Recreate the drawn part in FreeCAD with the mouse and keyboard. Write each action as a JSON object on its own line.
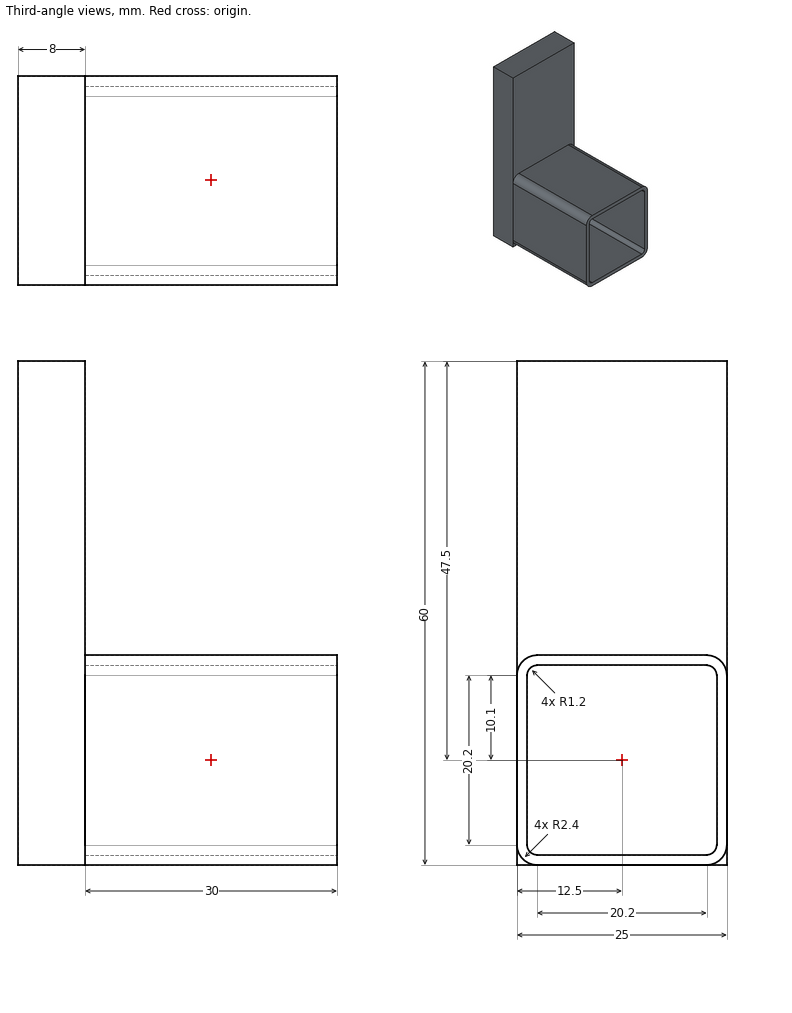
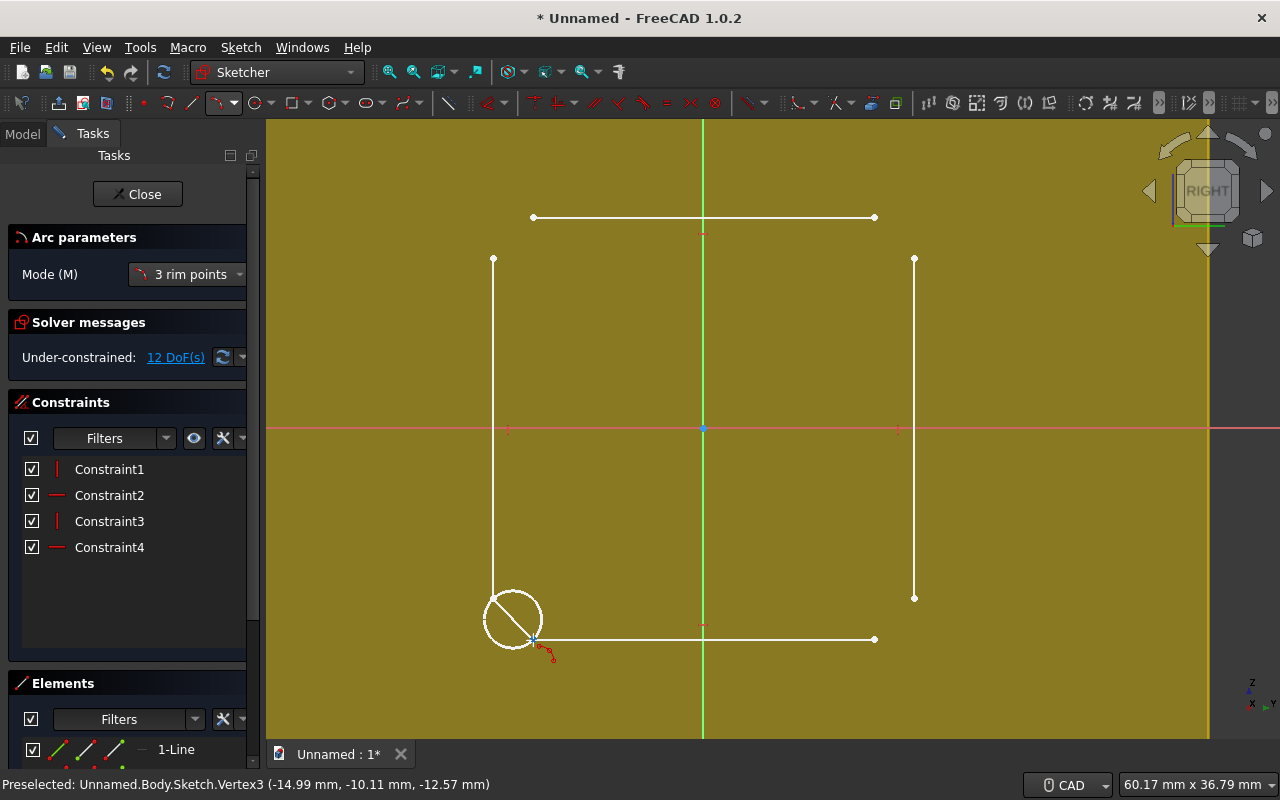
{"action": "scroll", "coordinate": [505, 627], "scroll_direction": "up", "scroll_amount": 2}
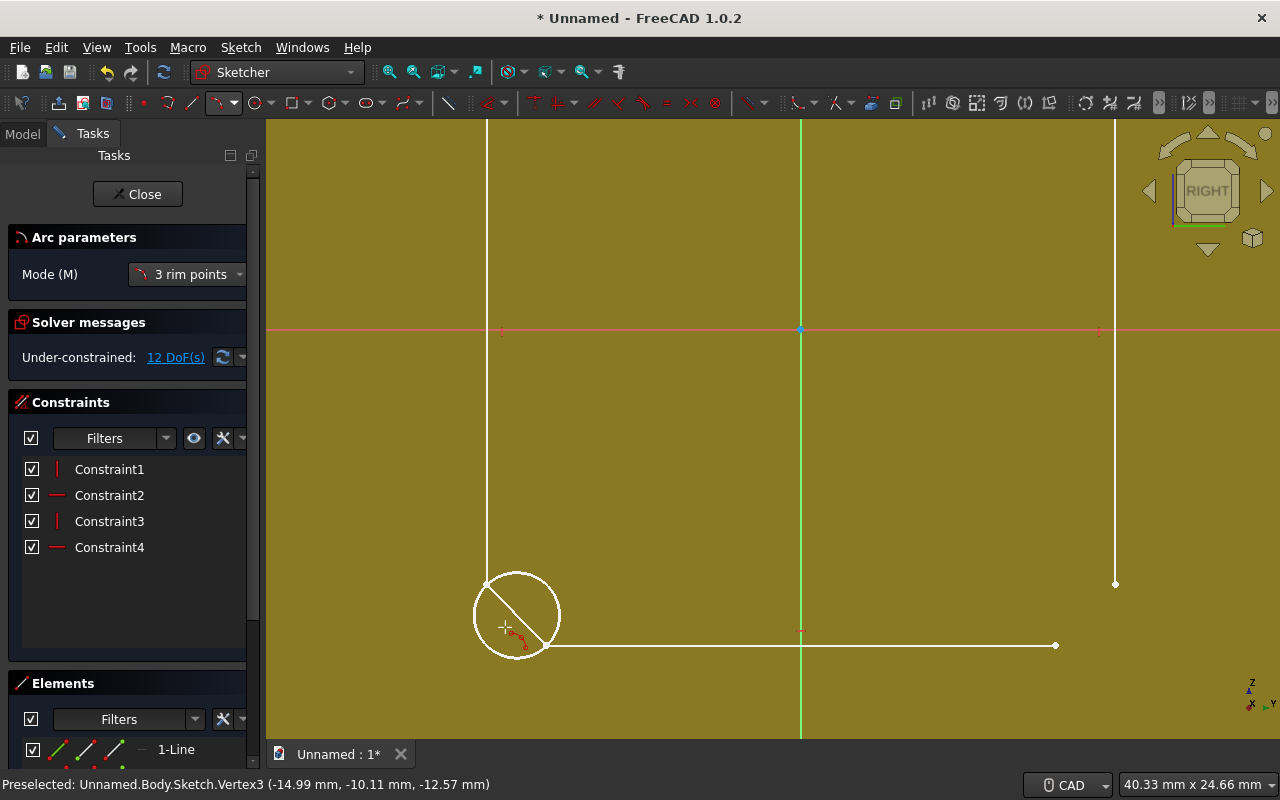
{"action": "left_click", "coordinate": [504, 627]}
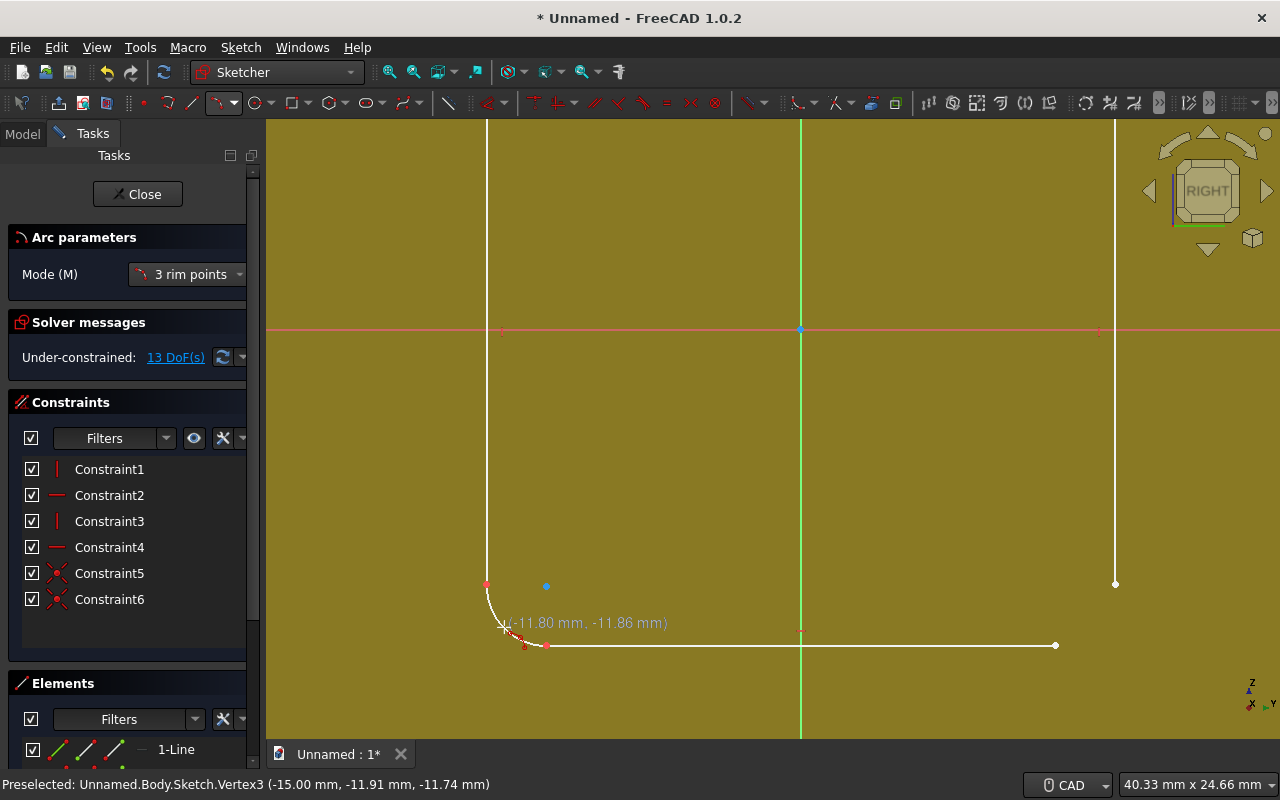
{"action": "left_click", "coordinate": [1055, 646]}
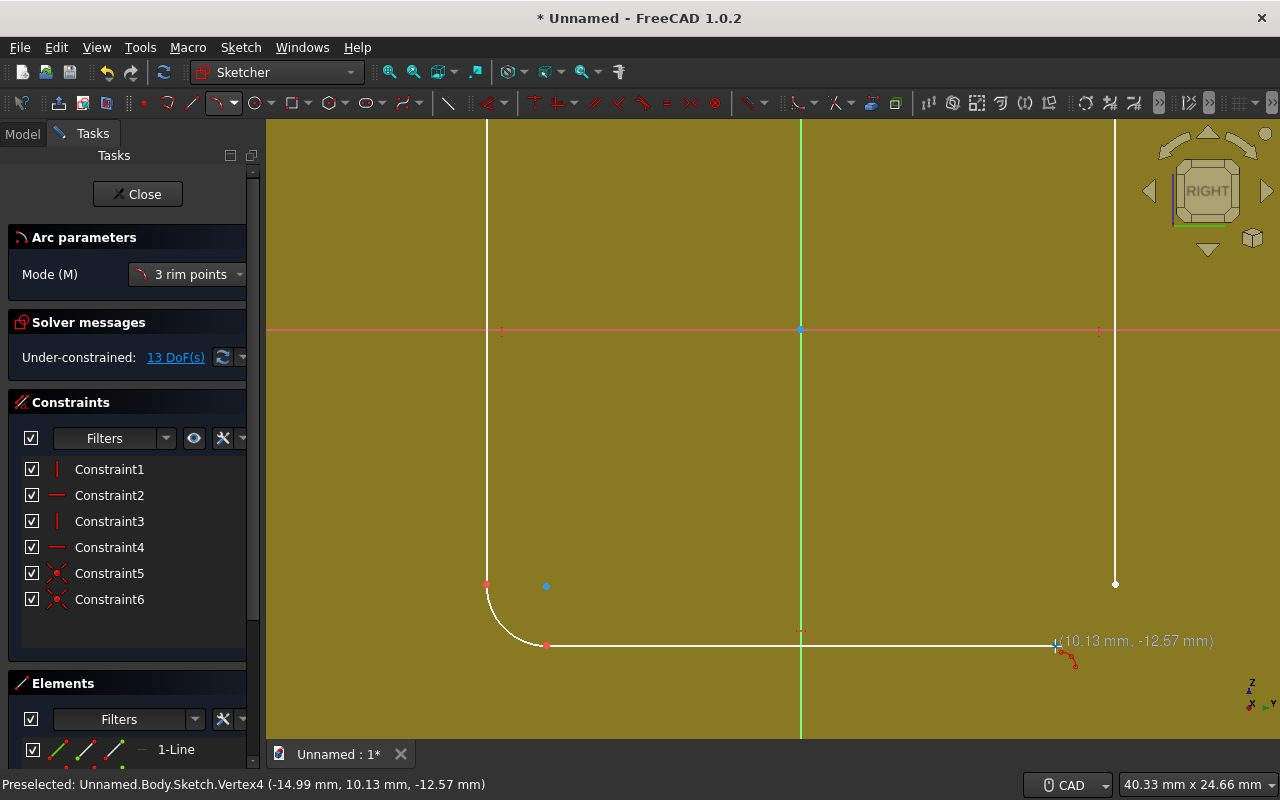
{"action": "scroll", "coordinate": [509, 630], "scroll_direction": "down", "scroll_amount": 2}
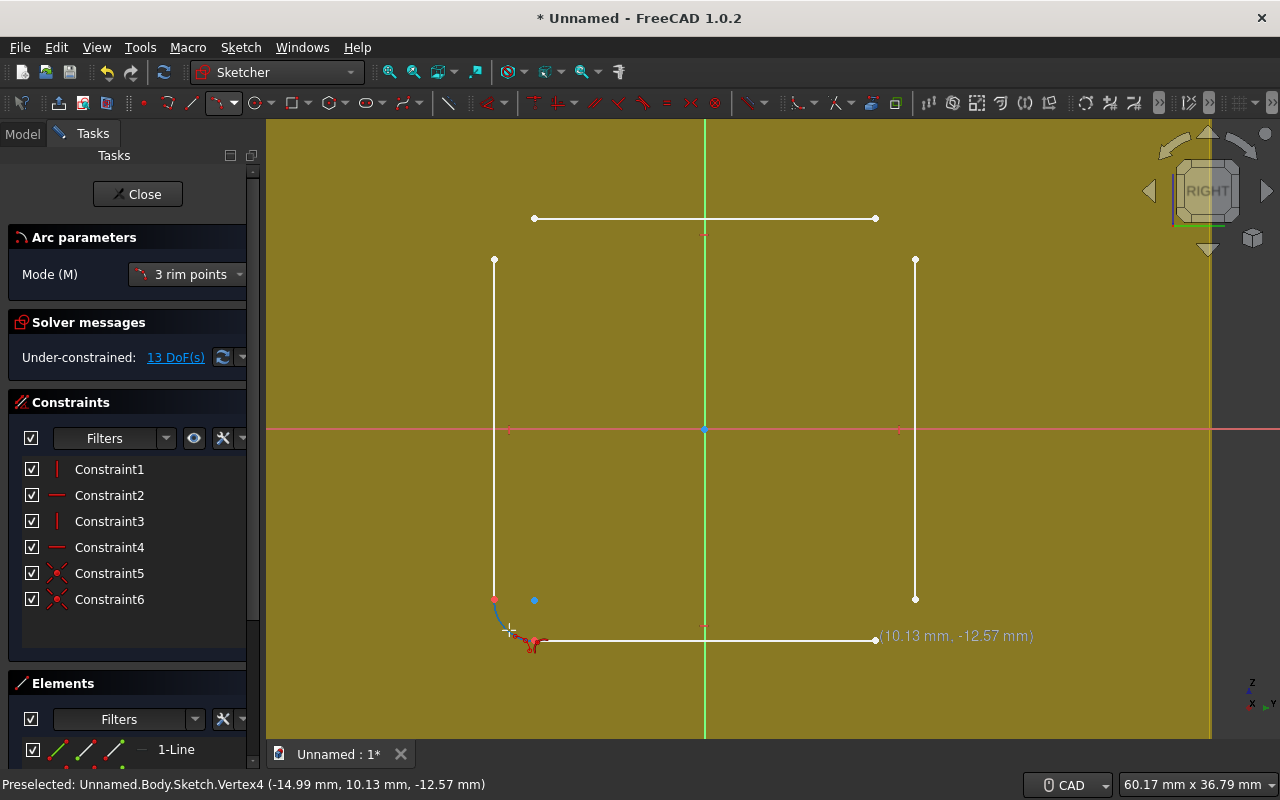
{"action": "left_click", "coordinate": [915, 600]}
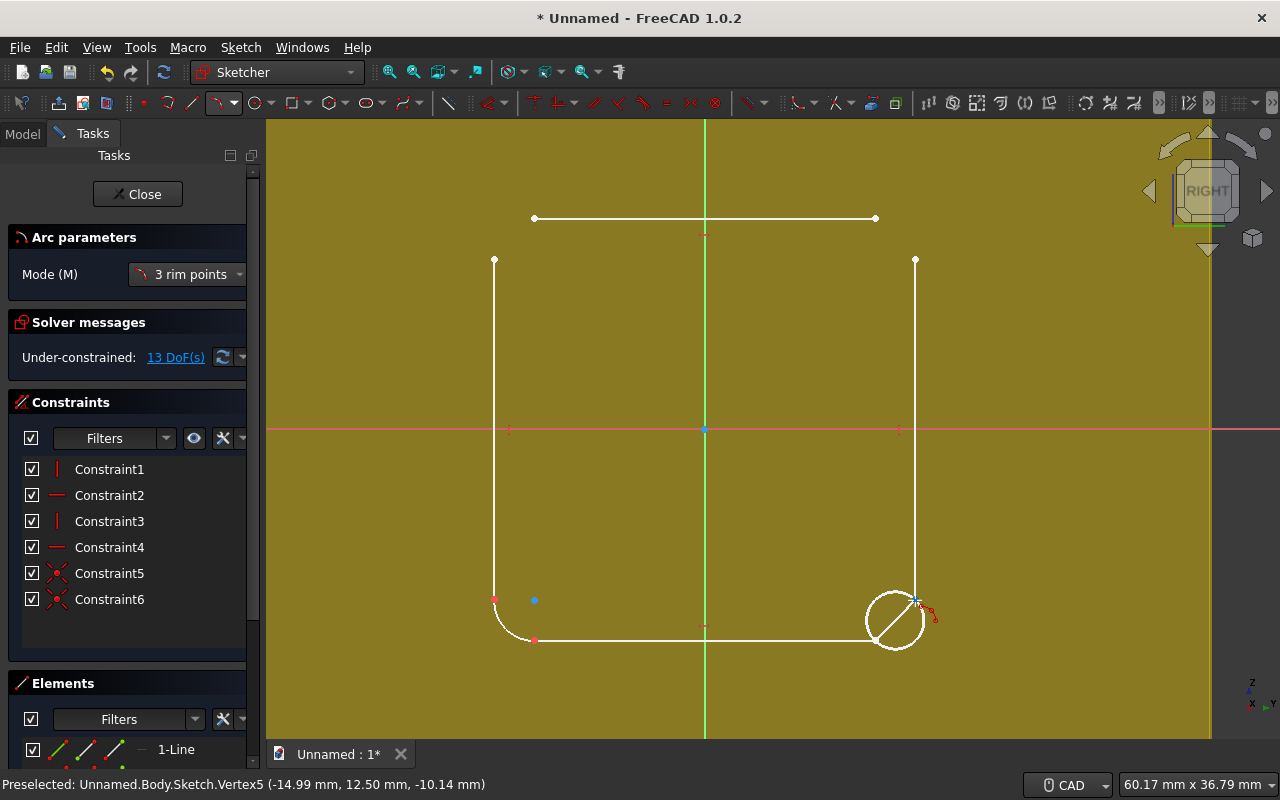
{"action": "scroll", "coordinate": [903, 628], "scroll_direction": "up", "scroll_amount": 2}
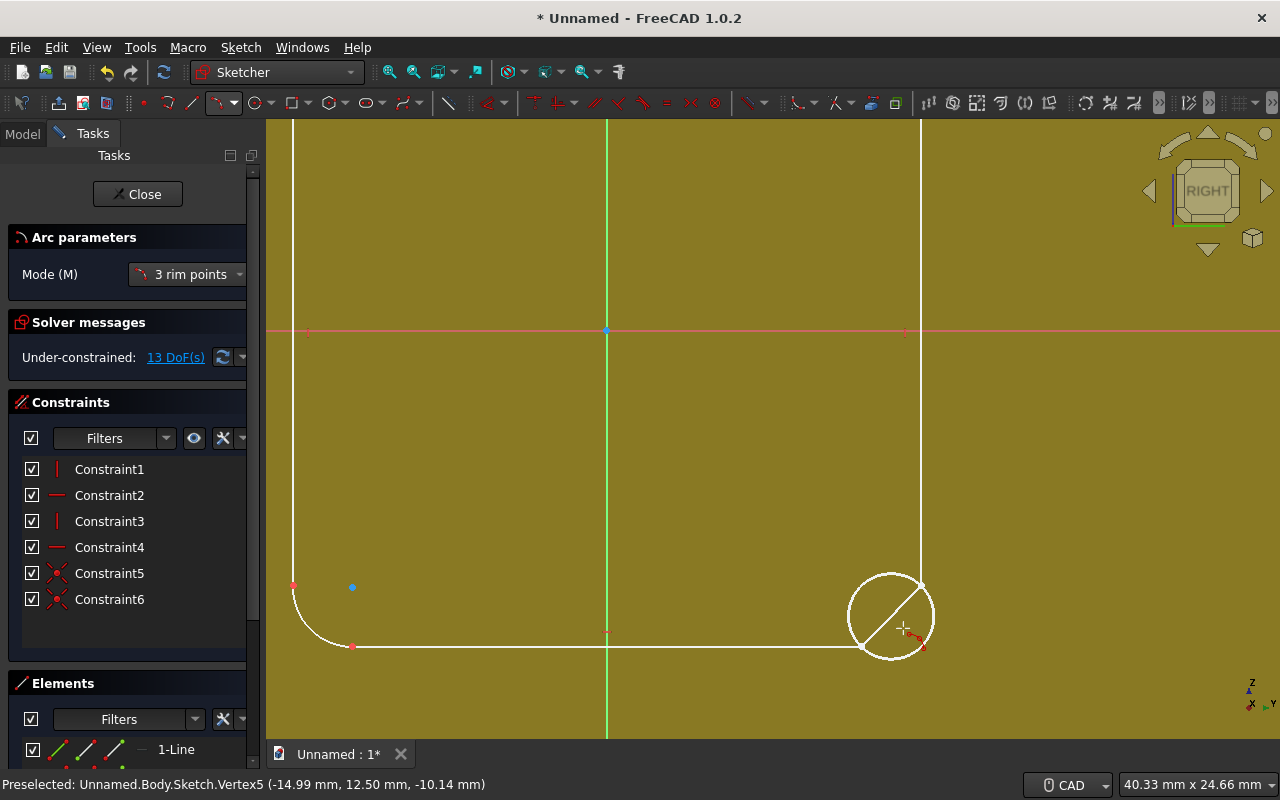
{"action": "left_click", "coordinate": [903, 628]}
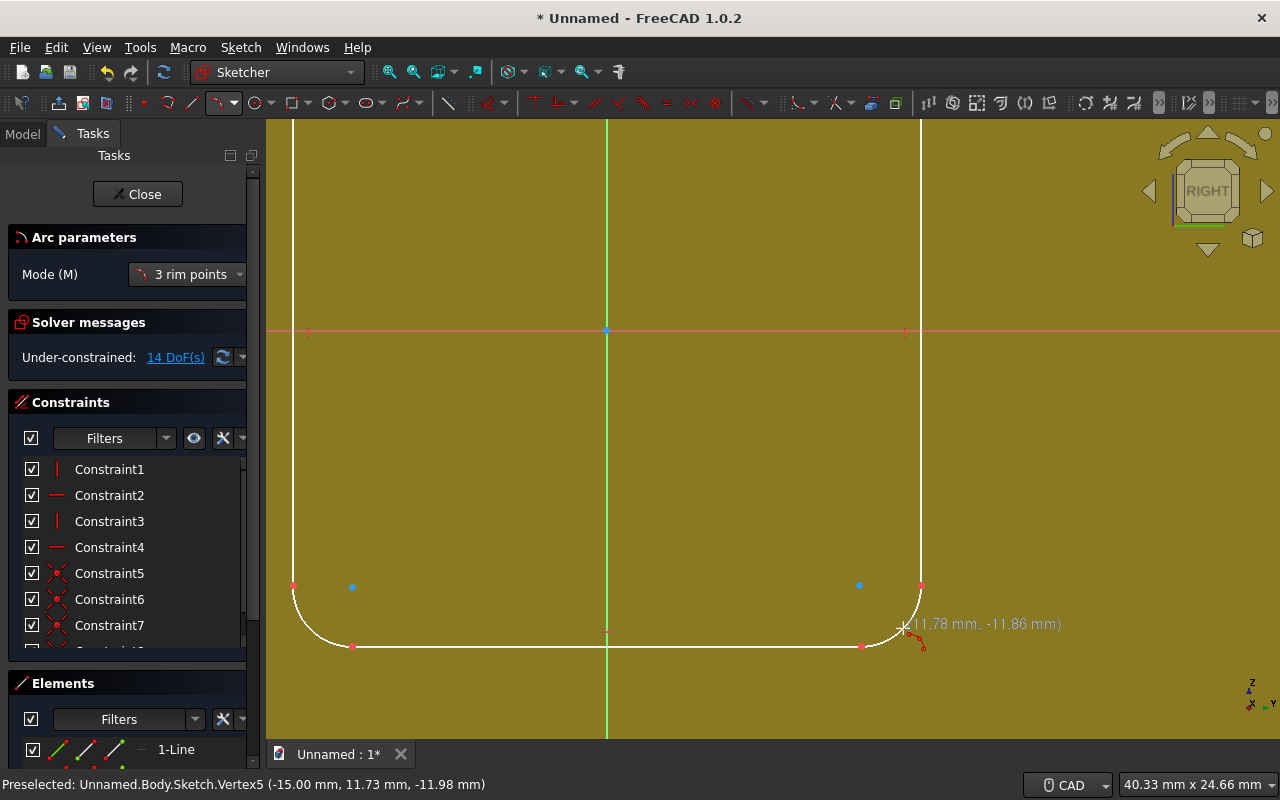
{"action": "scroll", "coordinate": [903, 628], "scroll_direction": "down", "scroll_amount": 2}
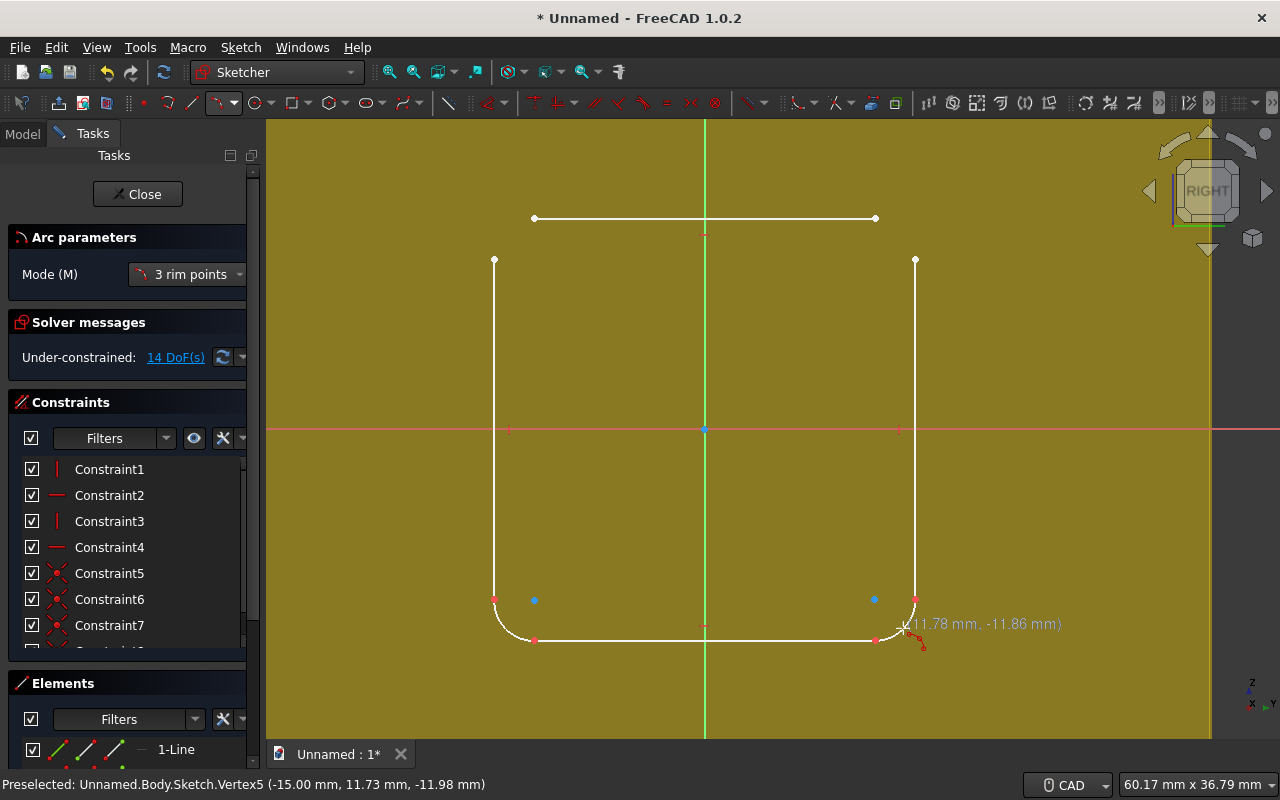
{"action": "left_click", "coordinate": [915, 260]}
{"action": "left_click", "coordinate": [875, 219]}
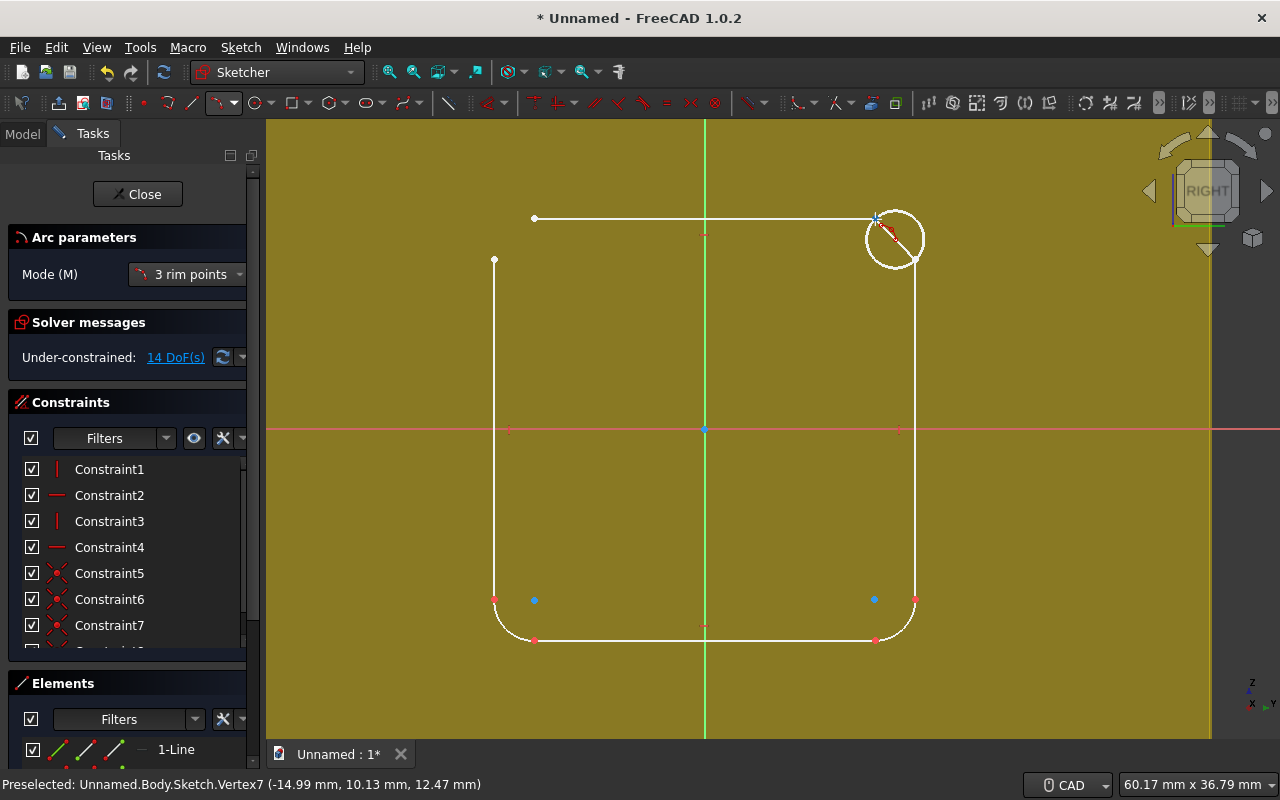
{"action": "scroll", "coordinate": [903, 230], "scroll_direction": "up", "scroll_amount": 2}